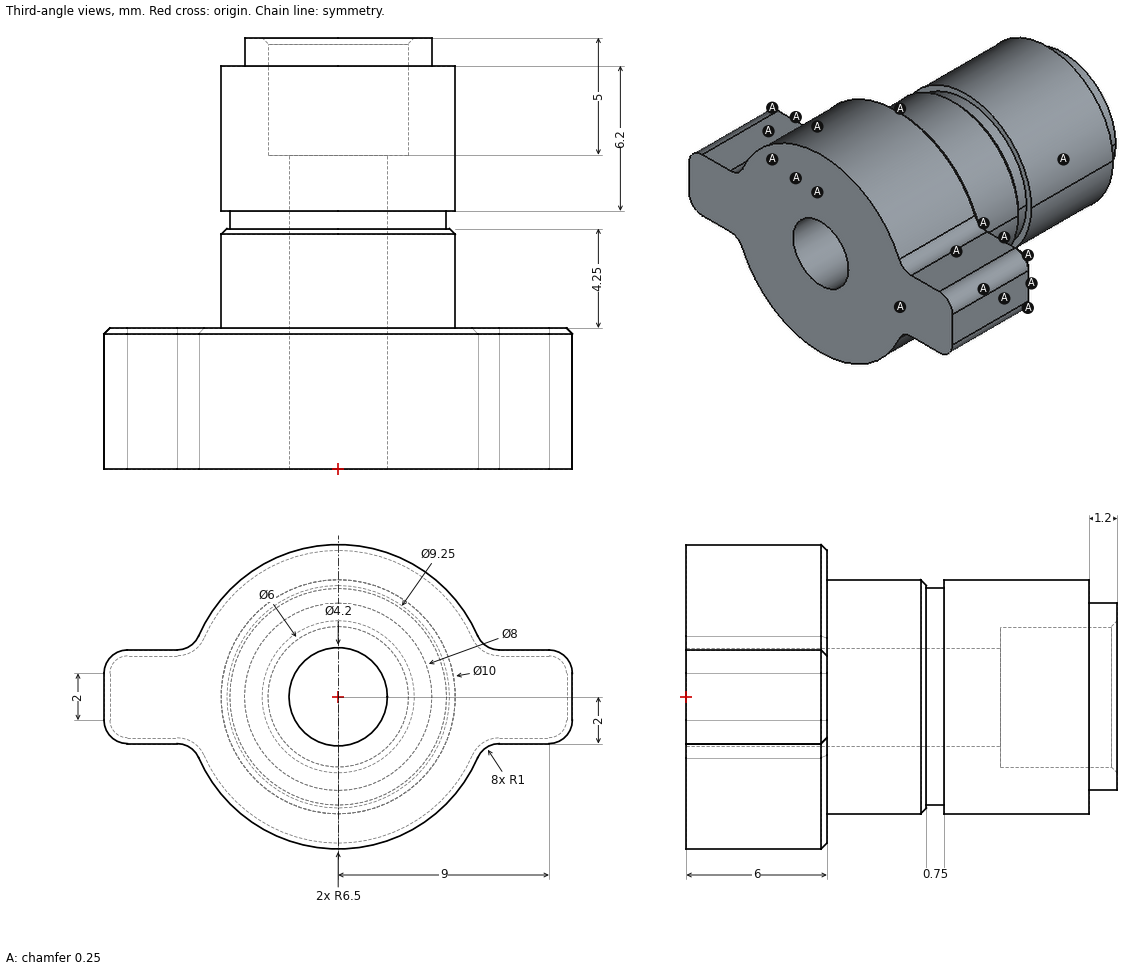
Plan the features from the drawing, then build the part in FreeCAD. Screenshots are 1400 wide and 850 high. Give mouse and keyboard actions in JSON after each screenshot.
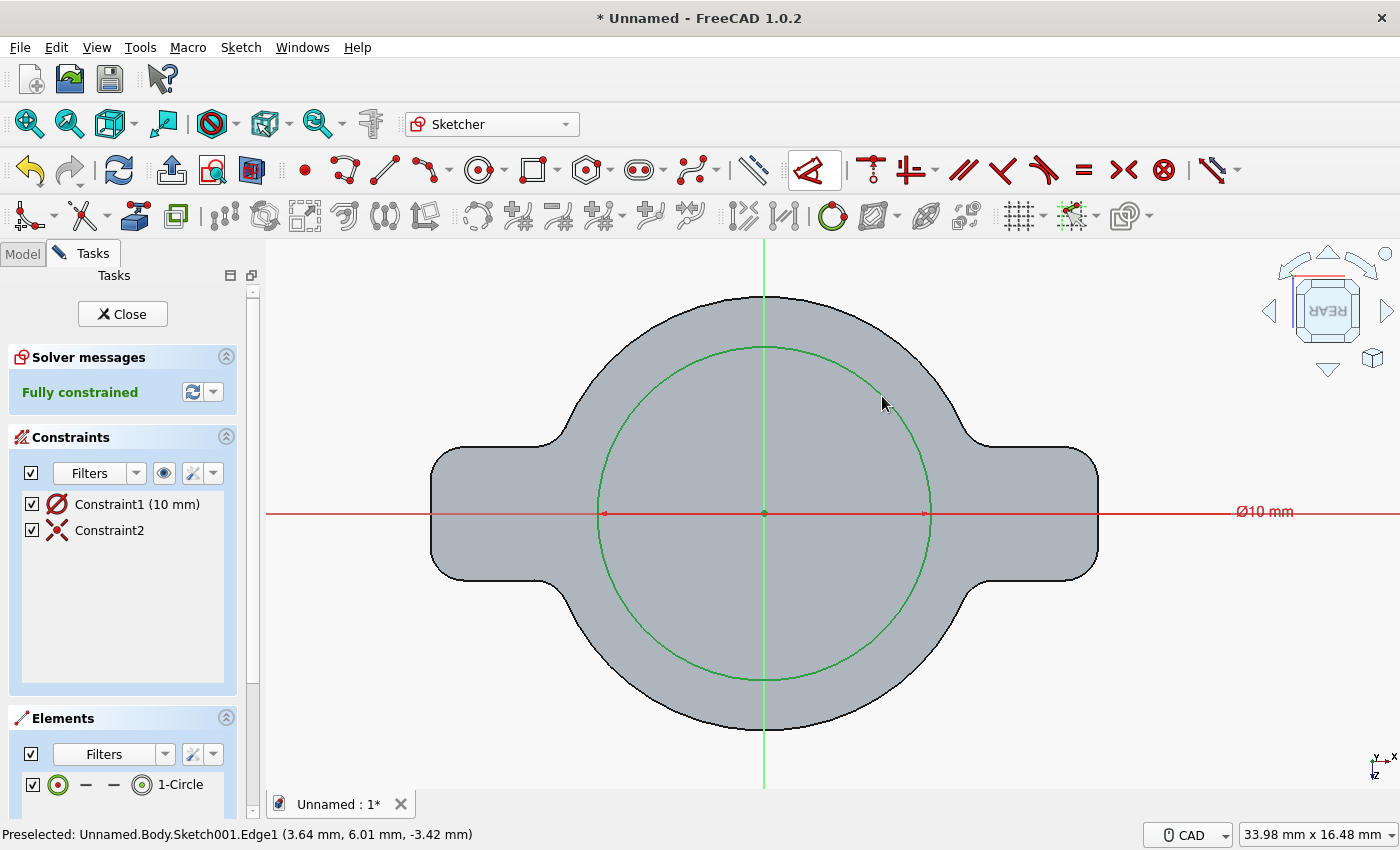
{"action": "left_click", "coordinate": [123, 314]}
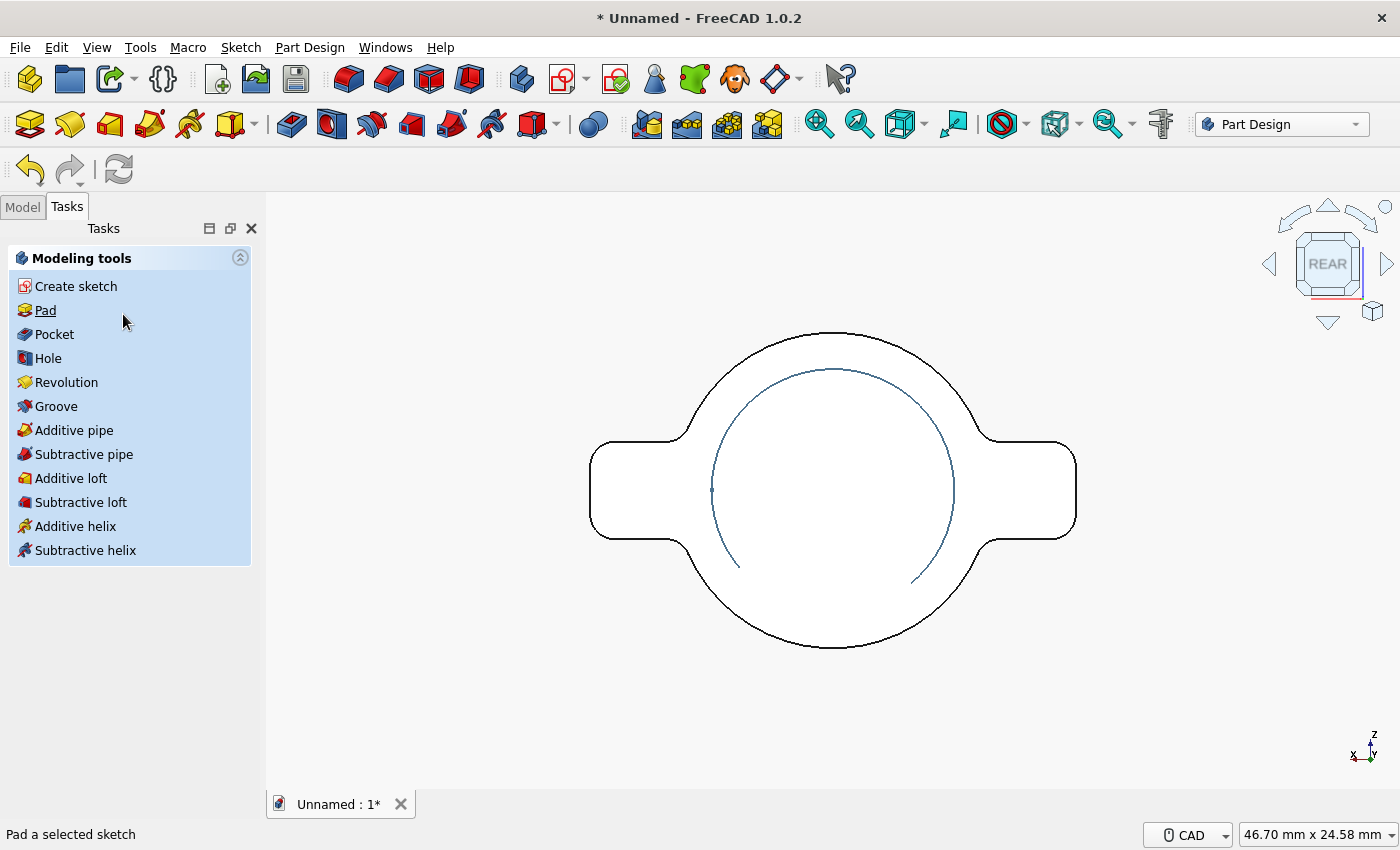
{"action": "left_click", "coordinate": [30, 124]}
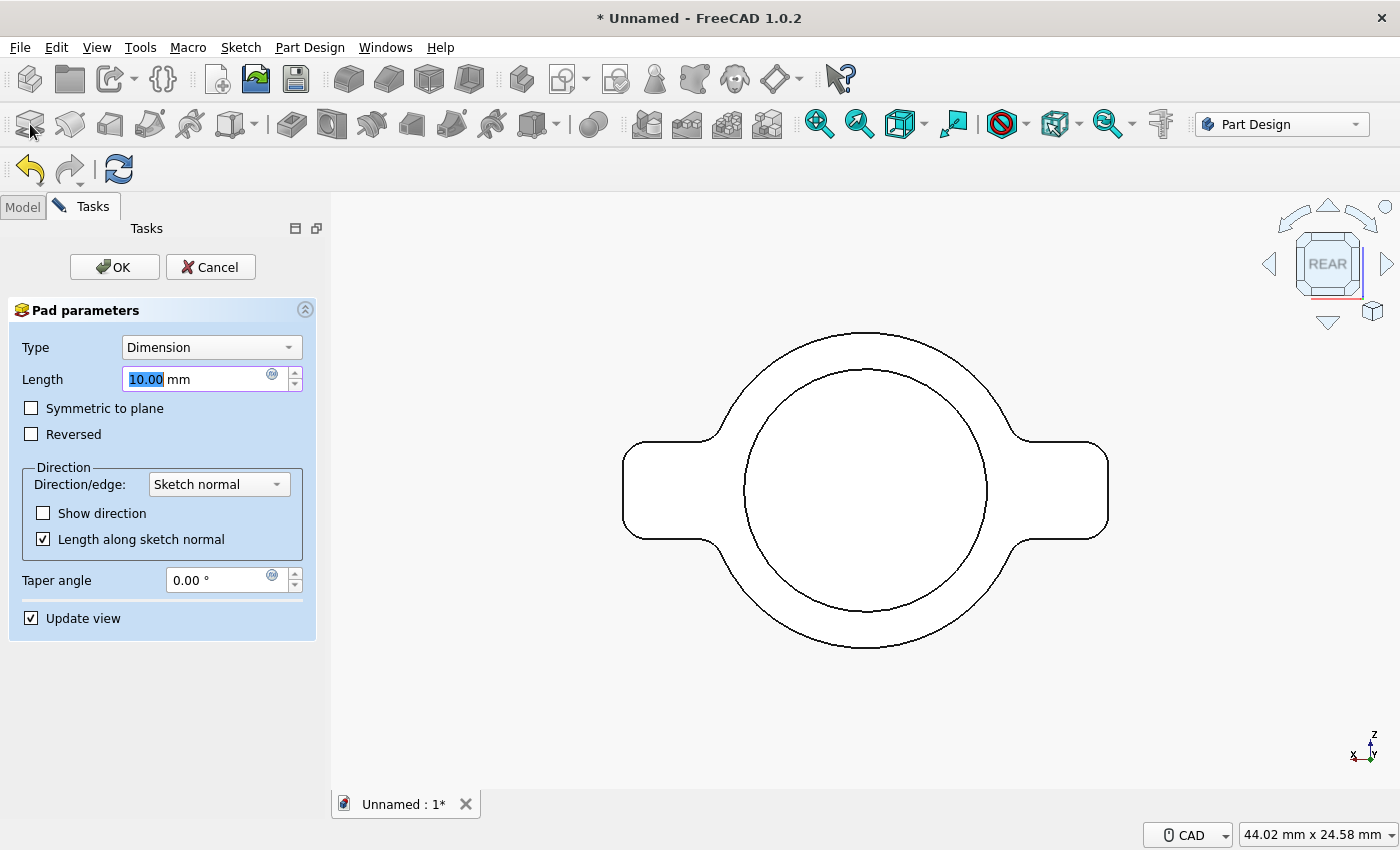
{"action": "type", "text": "4.25"}
{"action": "key", "text": "Tab"}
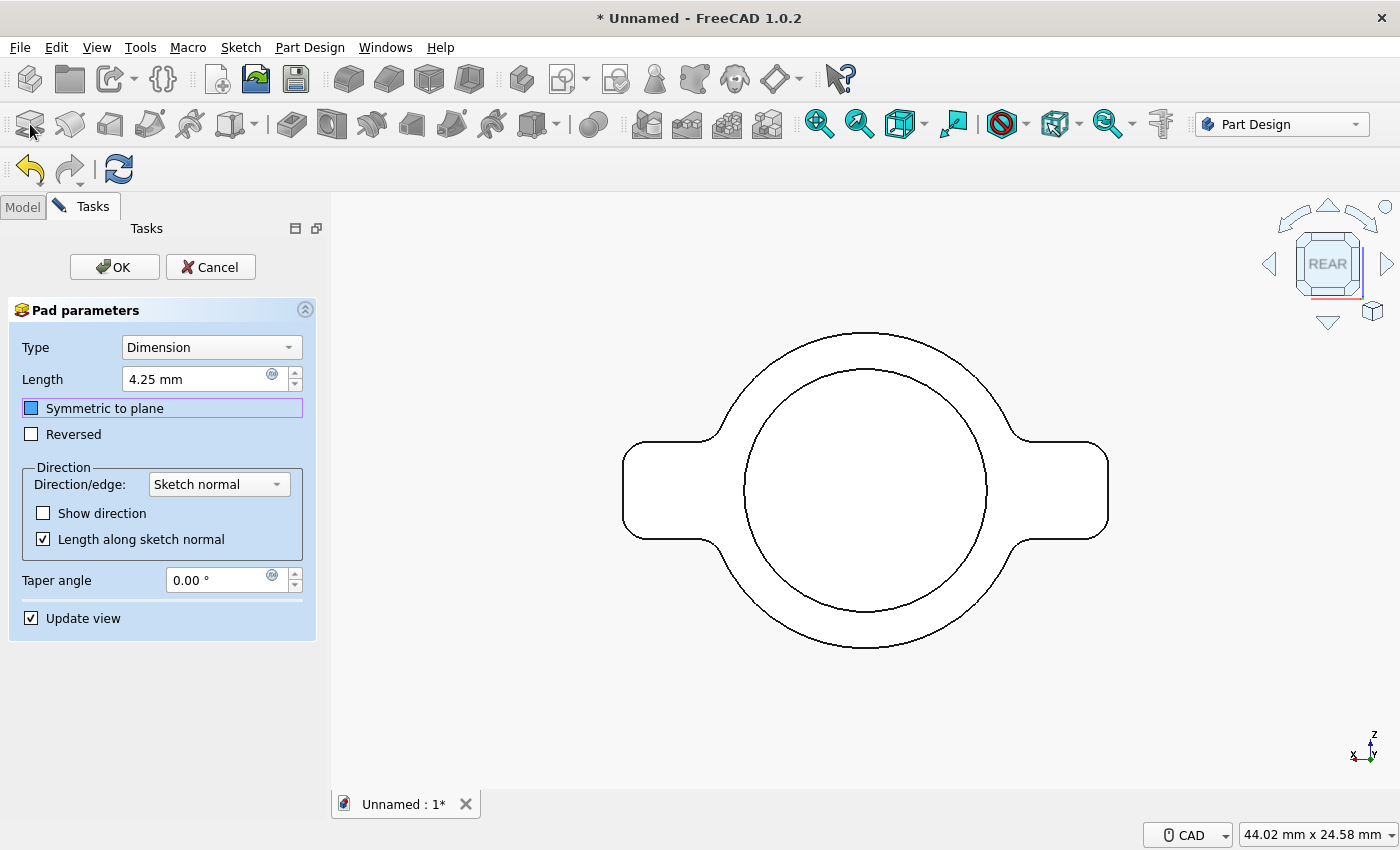
{"action": "left_click", "coordinate": [115, 267]}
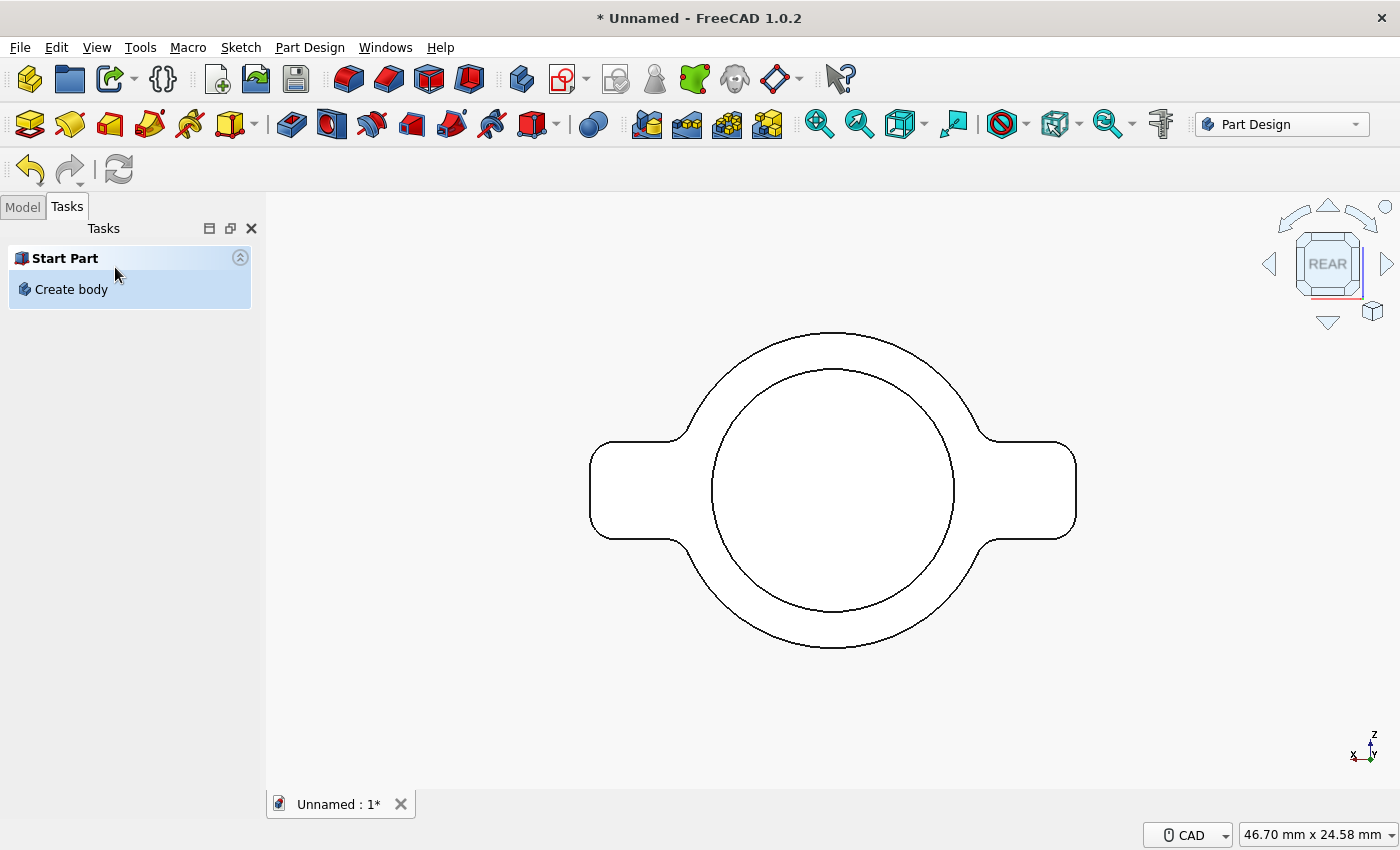
{"action": "left_click", "coordinate": [833, 490]}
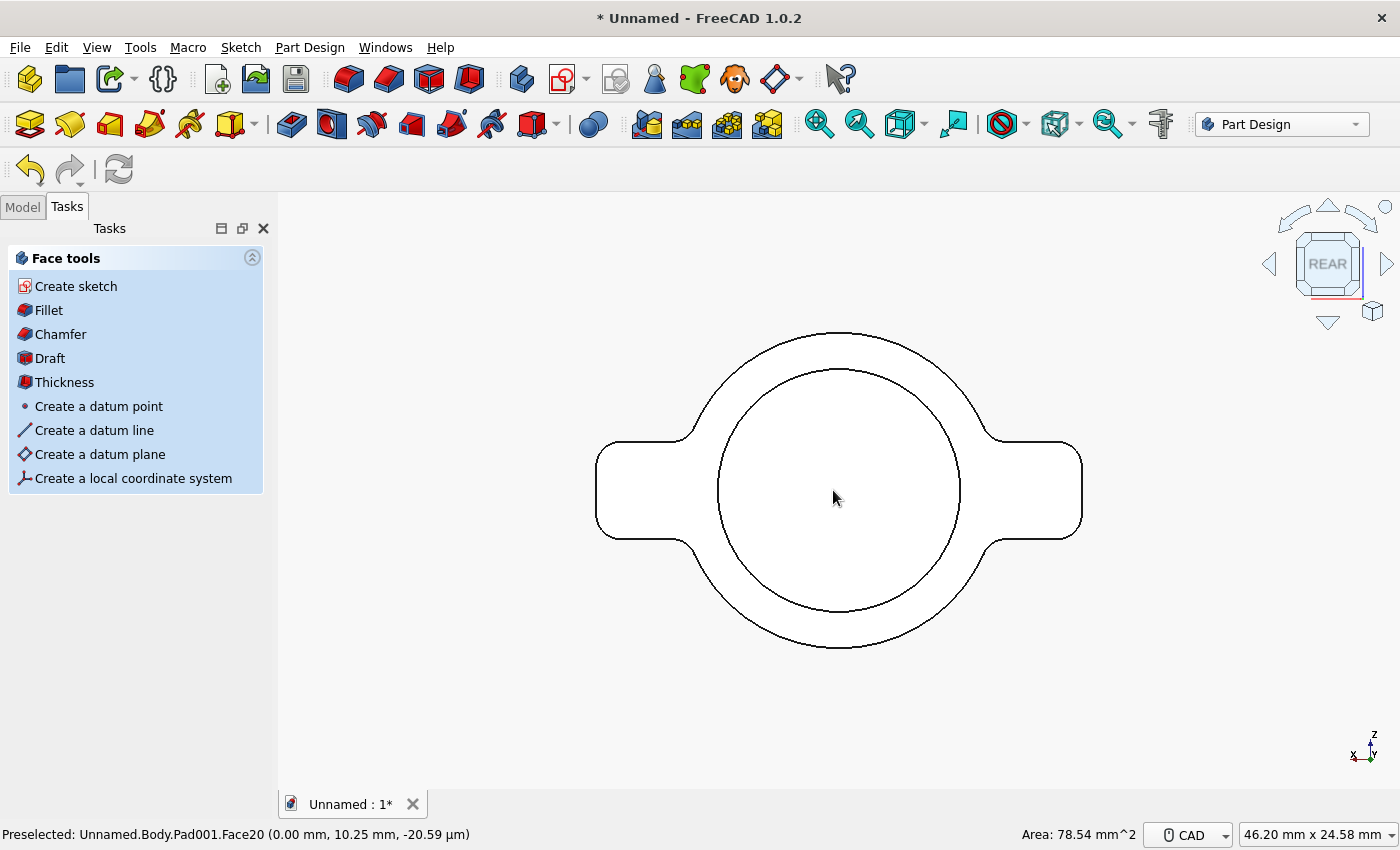
{"action": "left_click", "coordinate": [562, 80]}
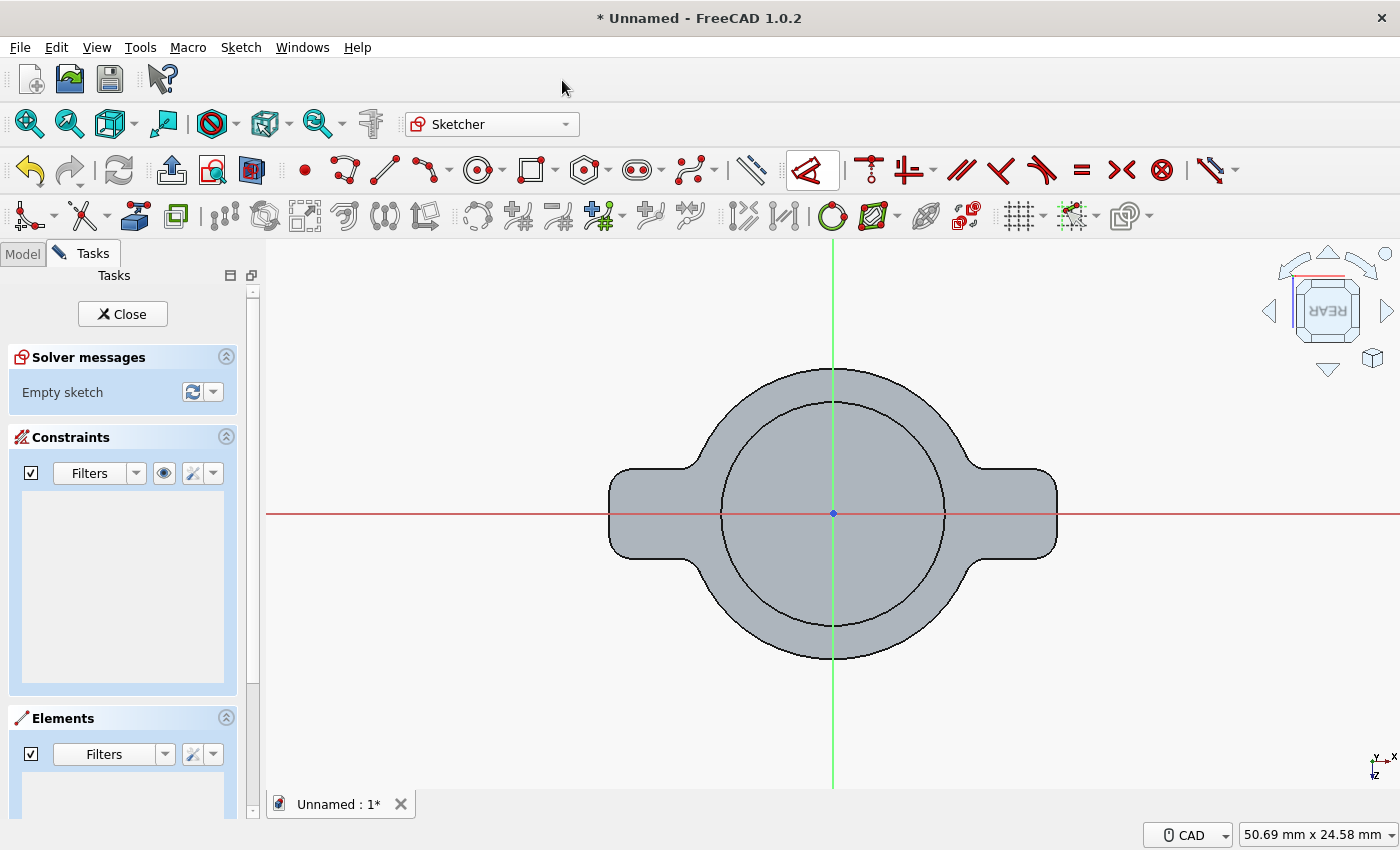
{"action": "scroll", "coordinate": [916, 514], "scroll_direction": "up", "scroll_amount": 3}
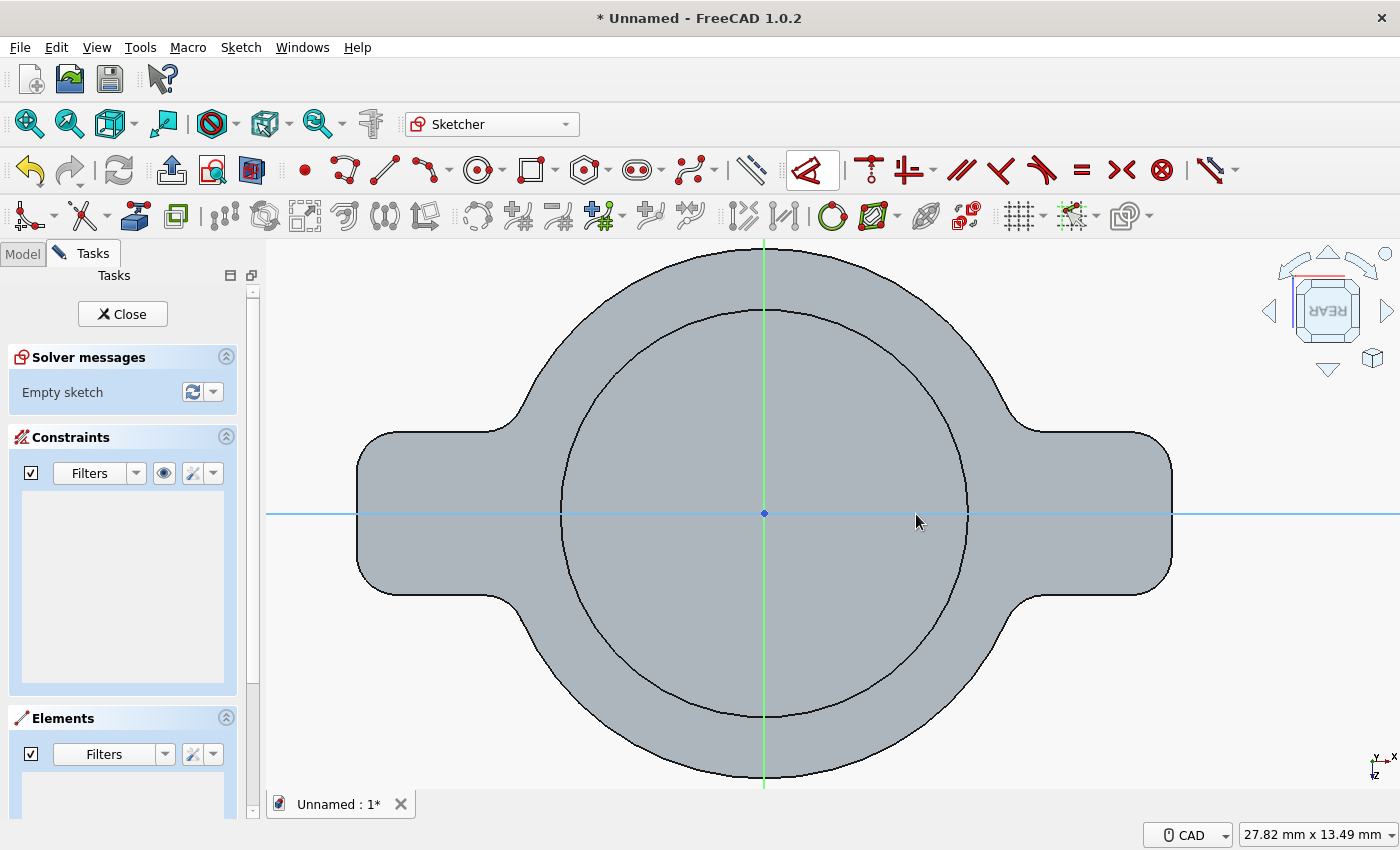
{"action": "left_click", "coordinate": [478, 170]}